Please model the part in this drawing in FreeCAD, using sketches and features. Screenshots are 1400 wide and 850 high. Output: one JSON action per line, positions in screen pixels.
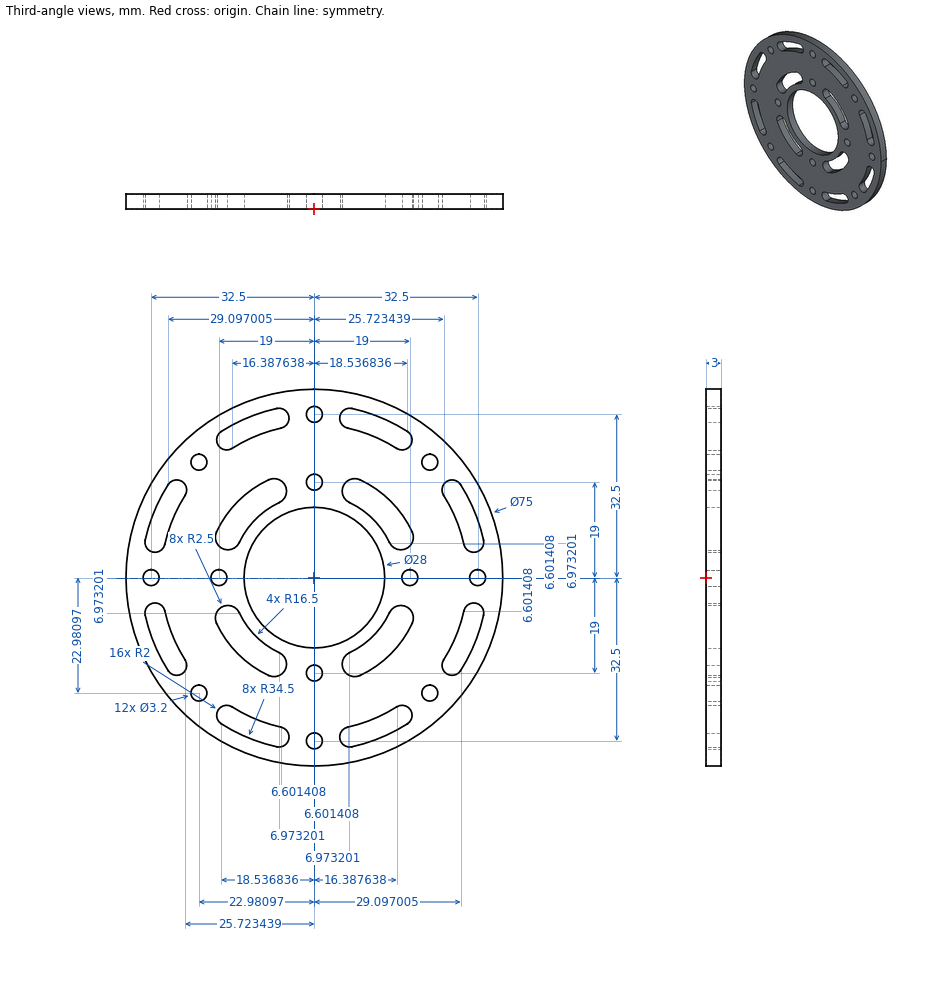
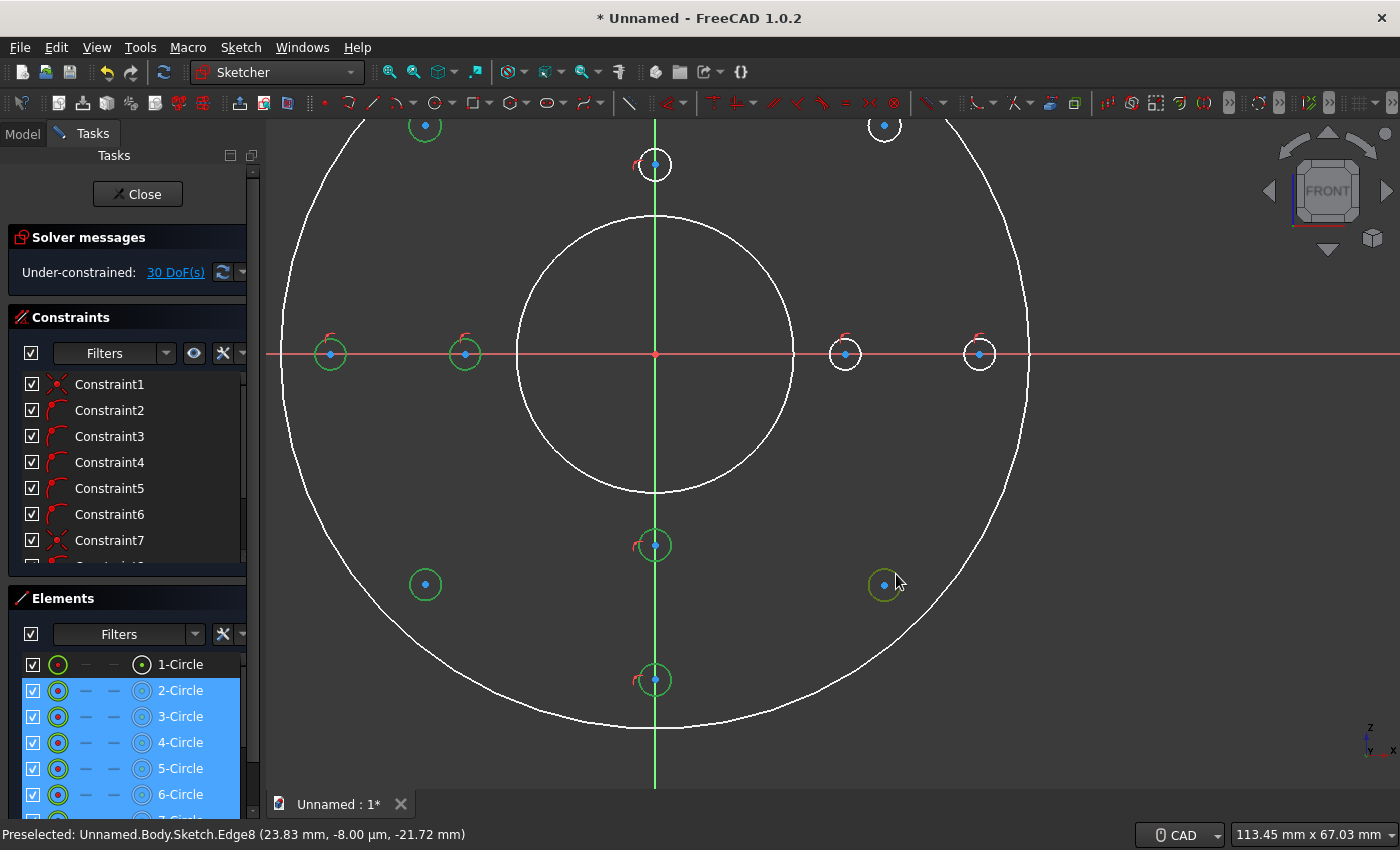
{"action": "scroll", "coordinate": [991, 343], "scroll_direction": "up", "scroll_amount": 2}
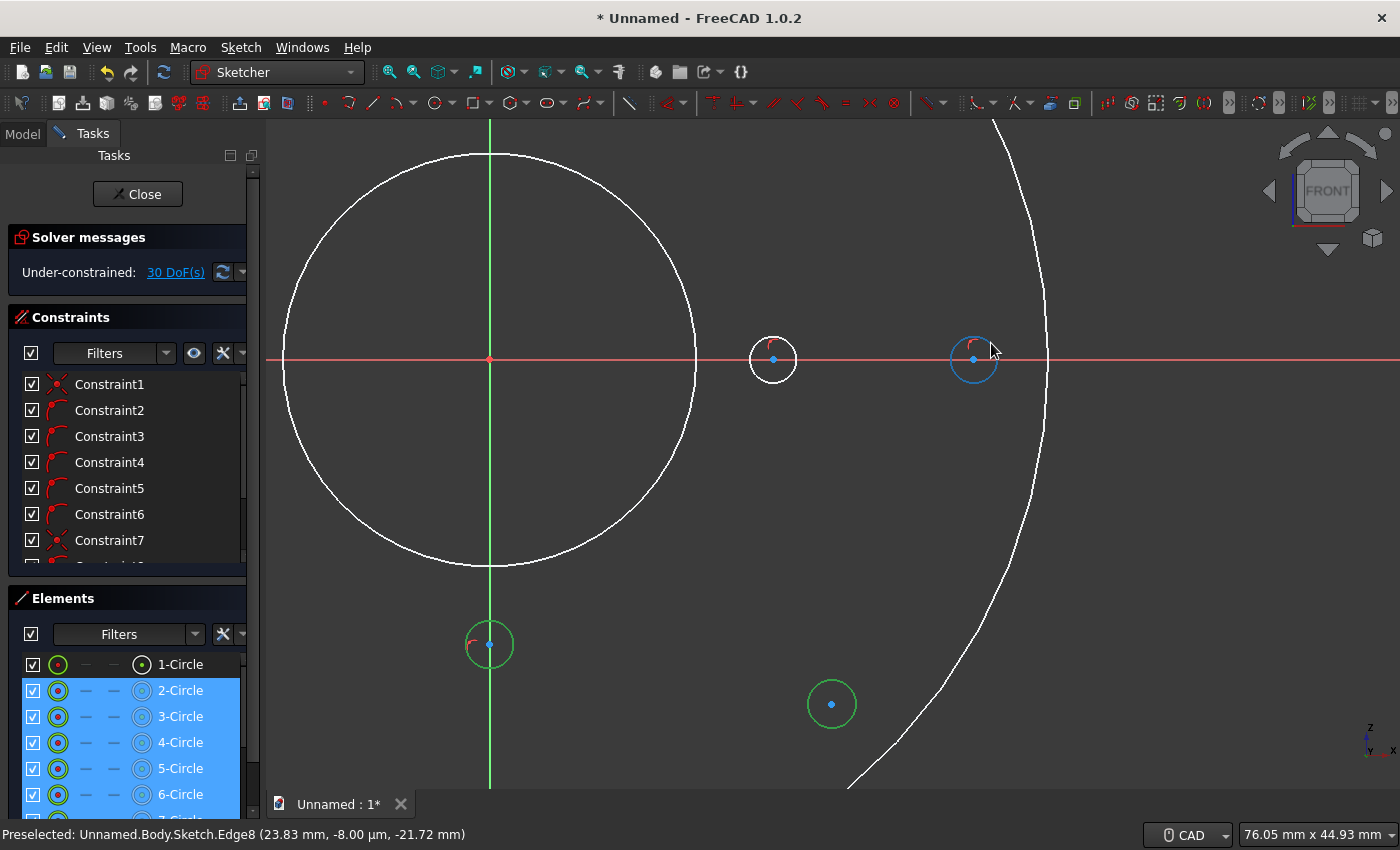
{"action": "left_click", "coordinate": [990, 343]}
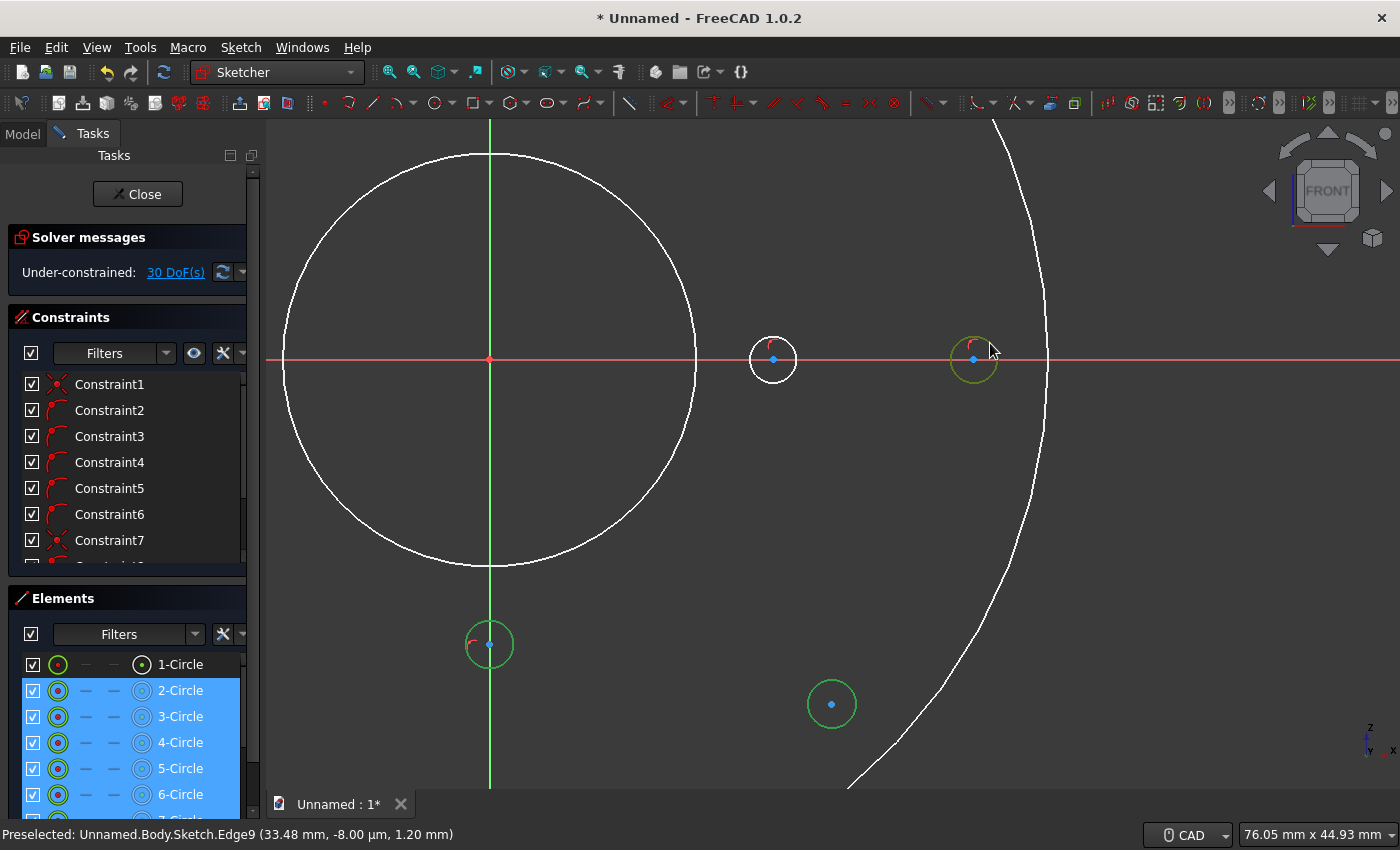
{"action": "scroll", "coordinate": [924, 509], "scroll_direction": "down", "scroll_amount": 5}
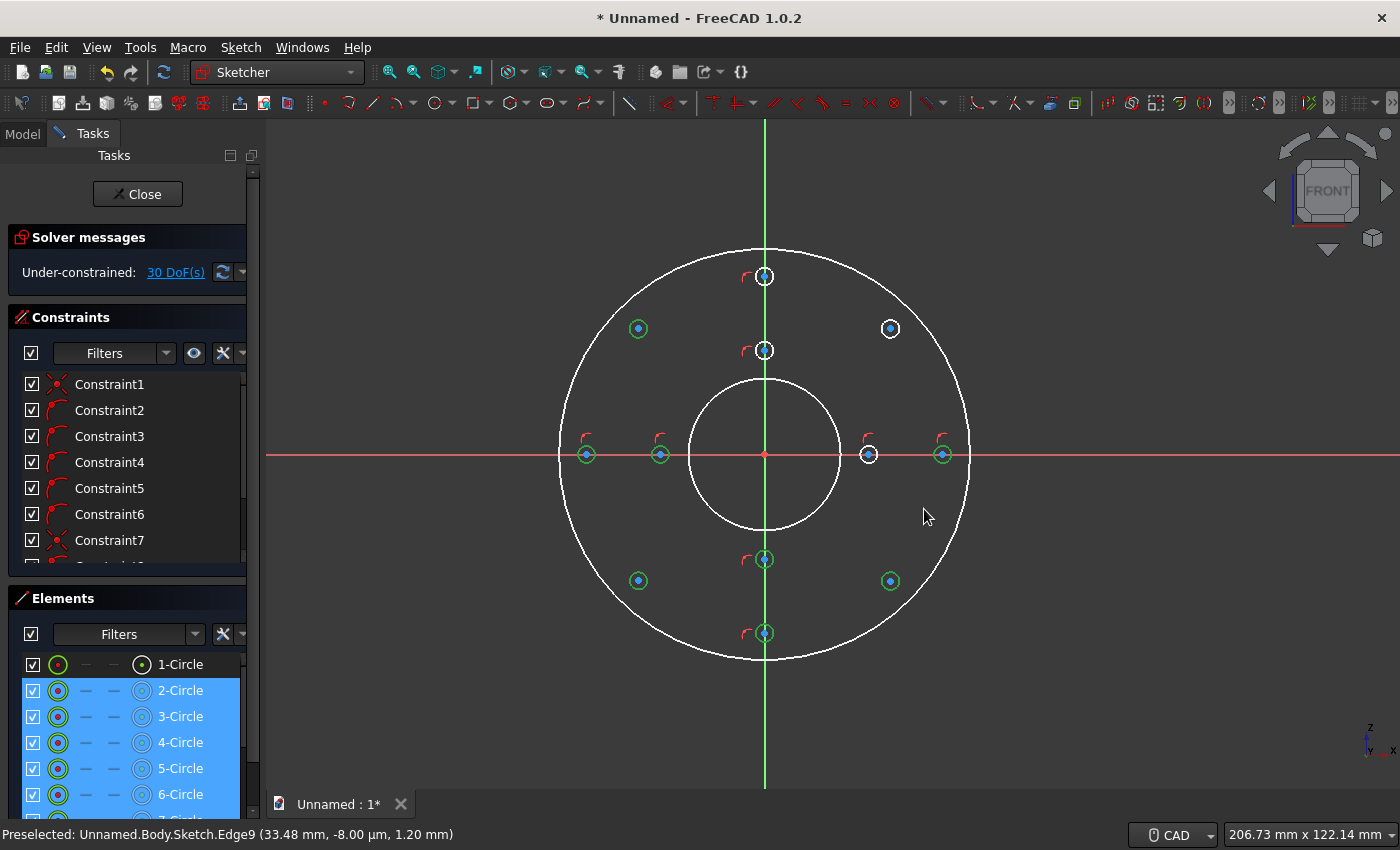
{"action": "scroll", "coordinate": [771, 344], "scroll_direction": "up", "scroll_amount": 5}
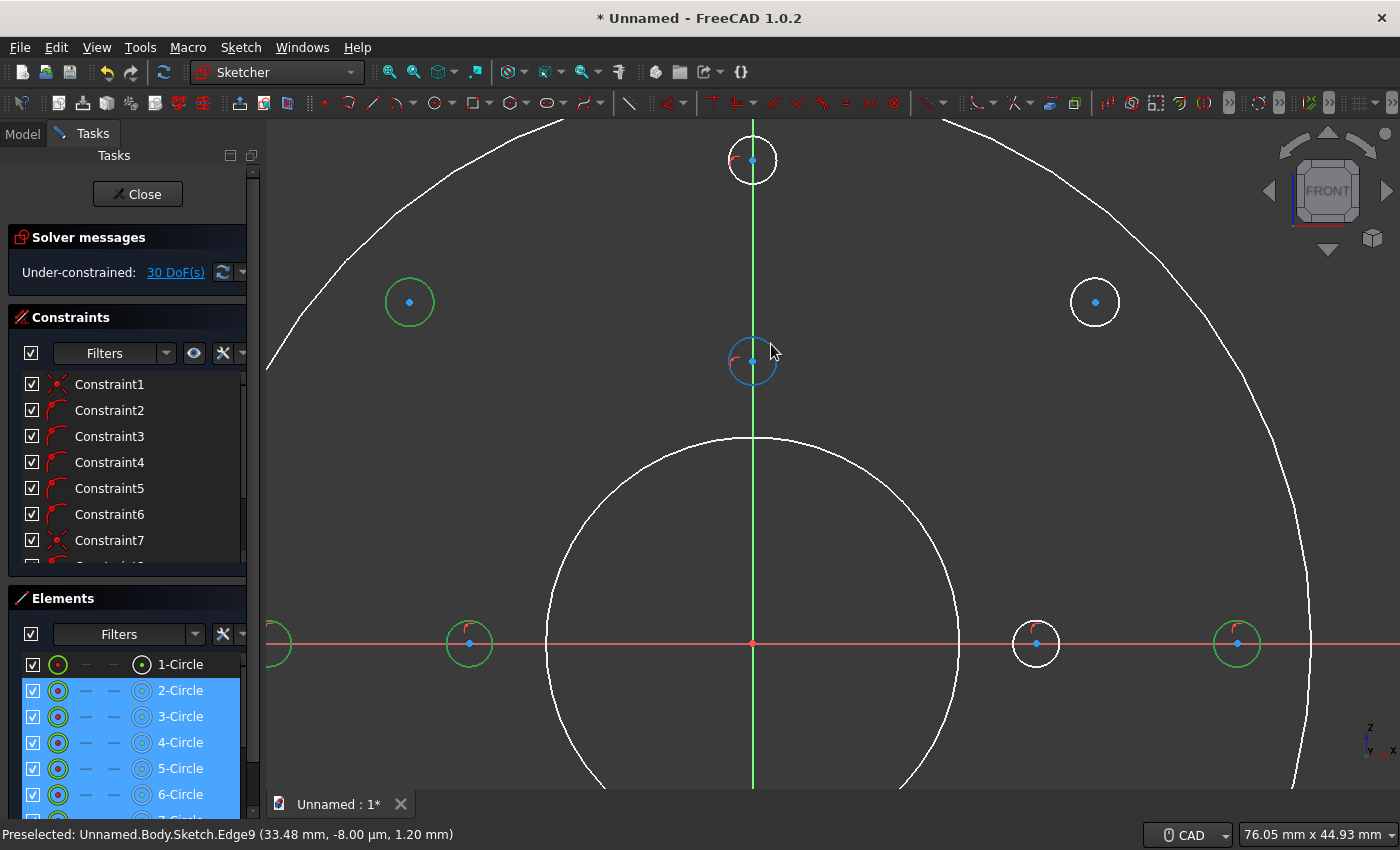
{"action": "left_click", "coordinate": [770, 344]}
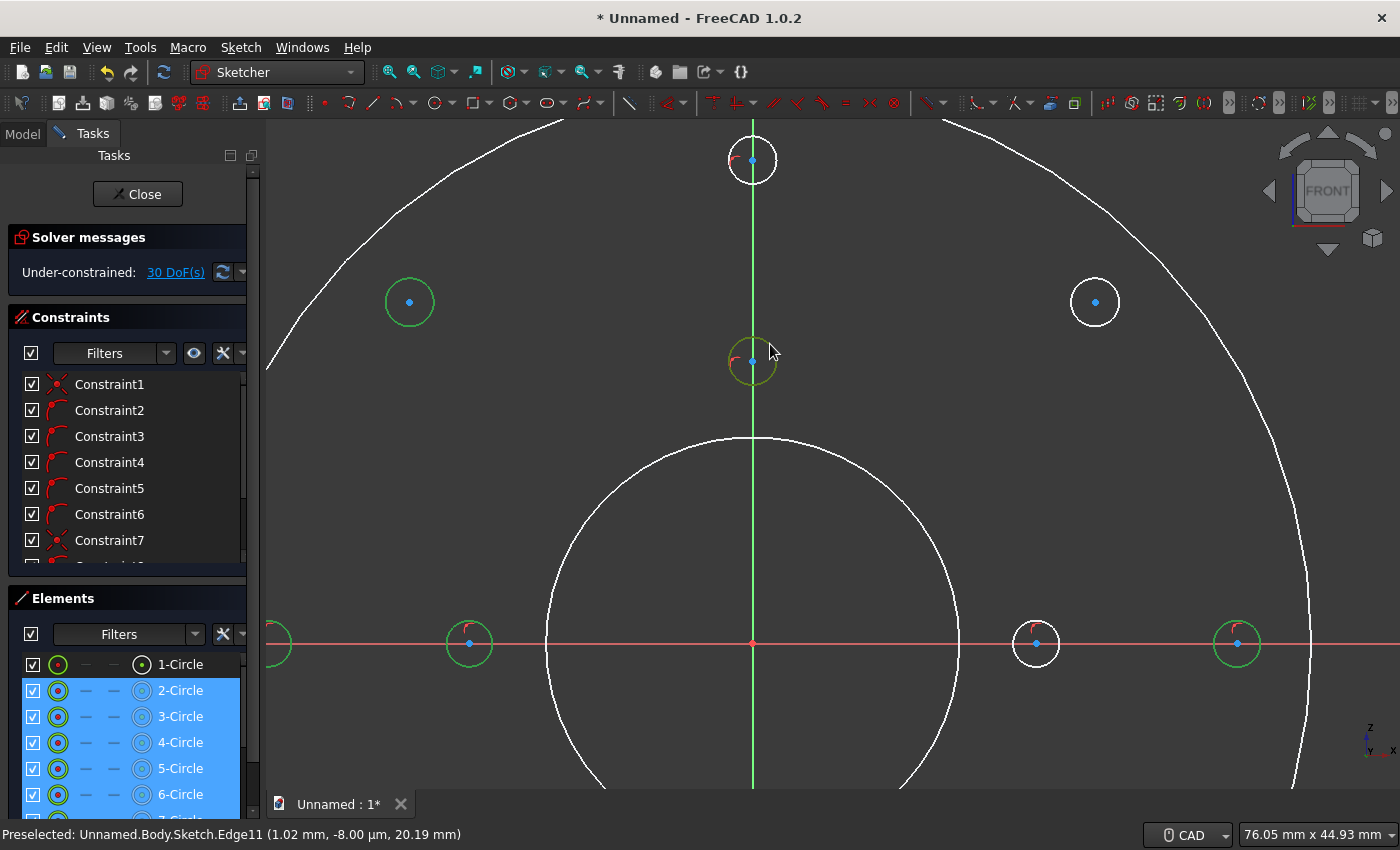
{"action": "left_click", "coordinate": [736, 177]}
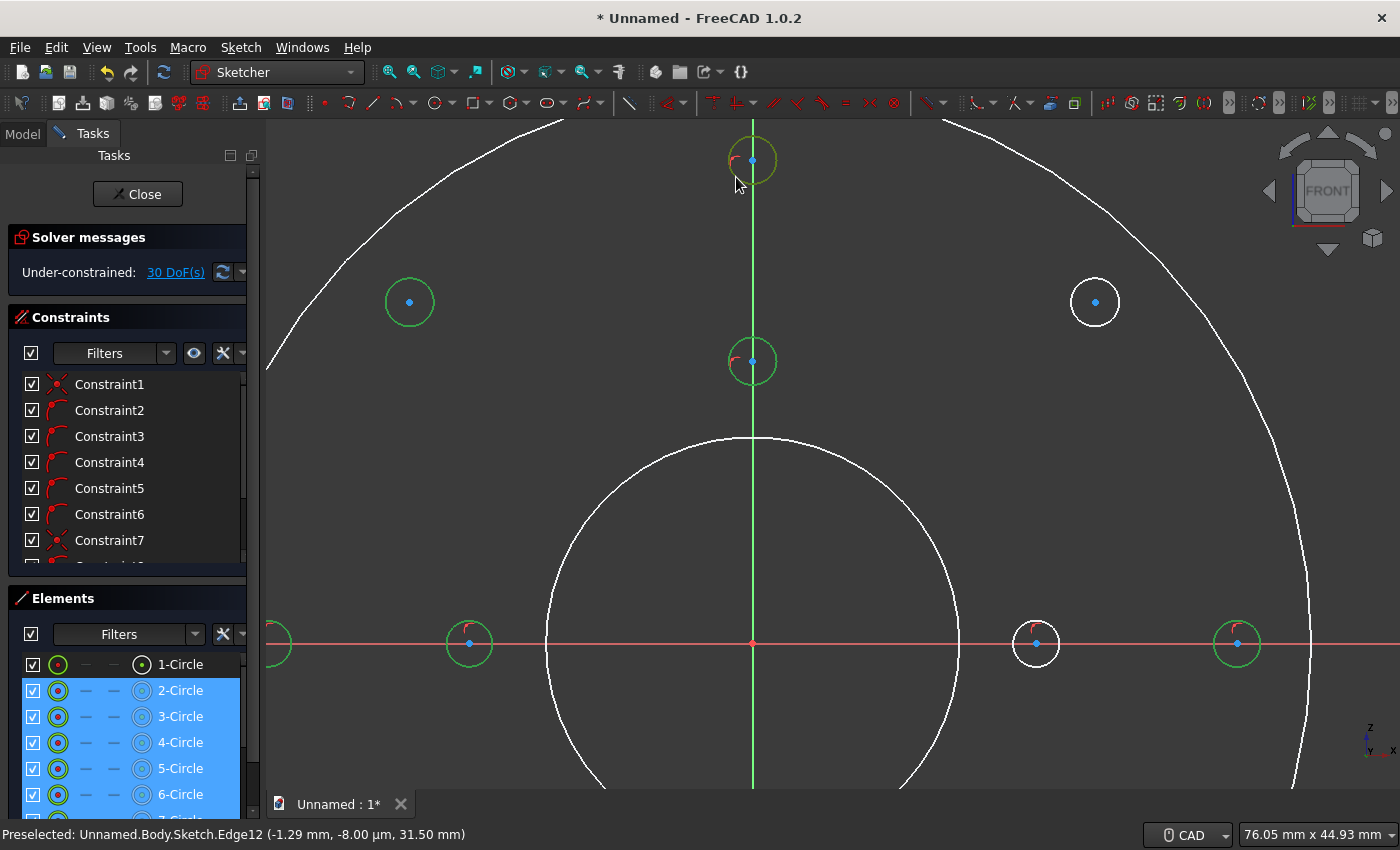
{"action": "left_click", "coordinate": [1053, 627]}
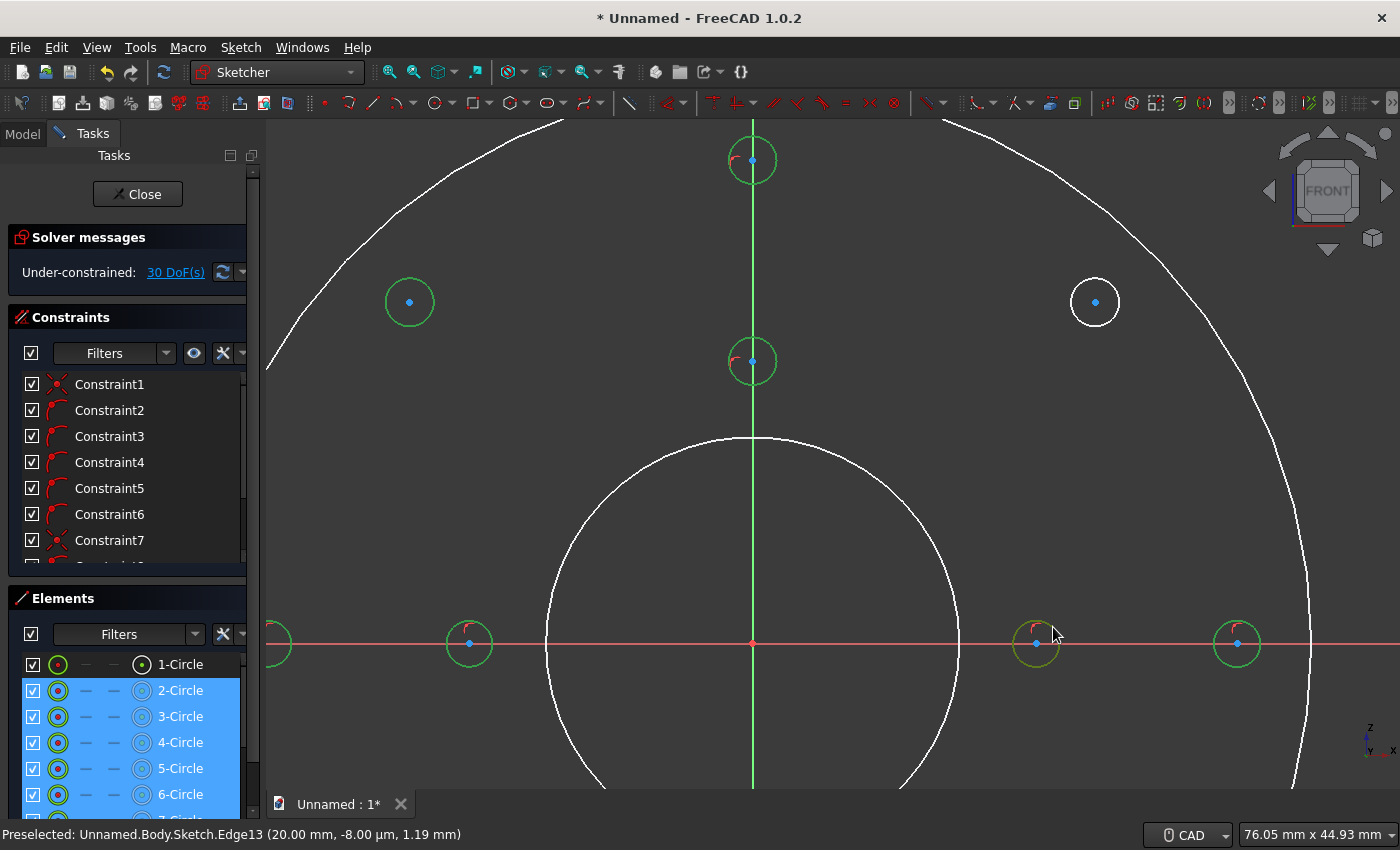
{"action": "left_click", "coordinate": [1112, 285]}